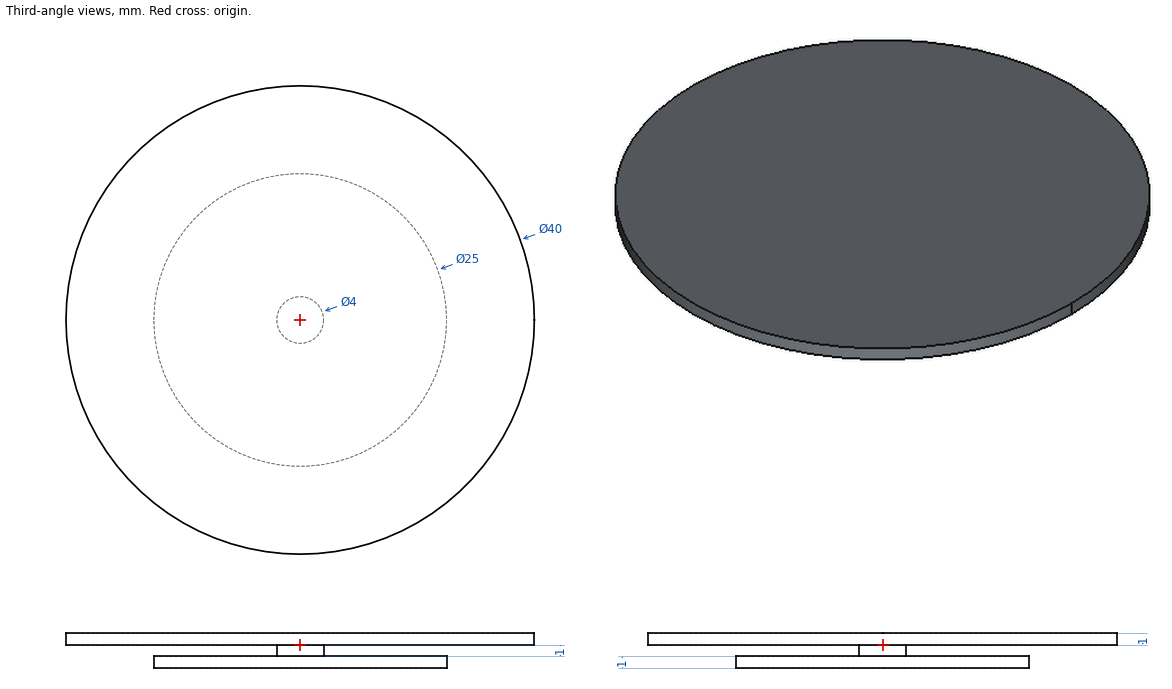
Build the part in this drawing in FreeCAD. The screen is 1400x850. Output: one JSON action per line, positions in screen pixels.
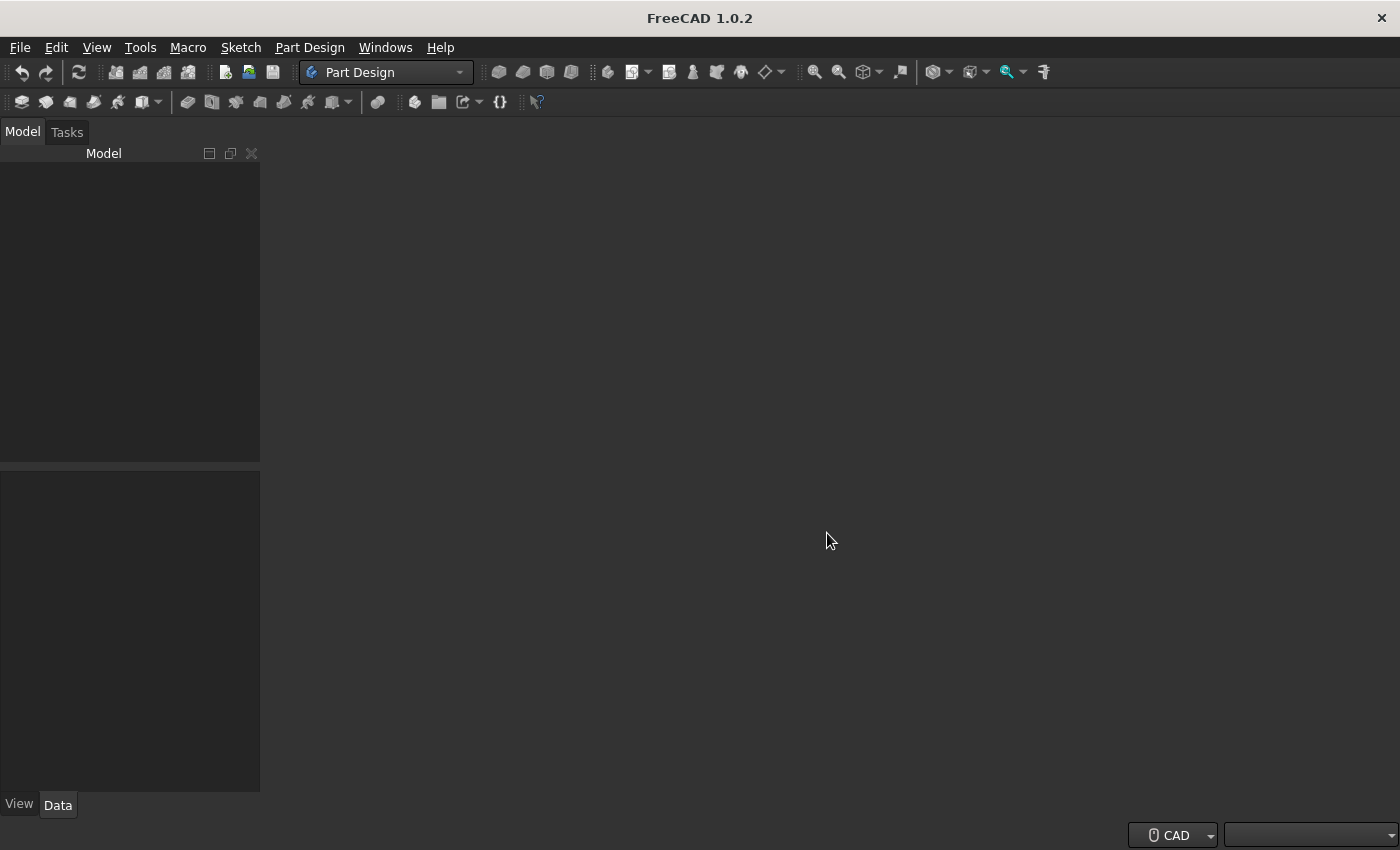
{"action": "key", "text": "ctrl+n"}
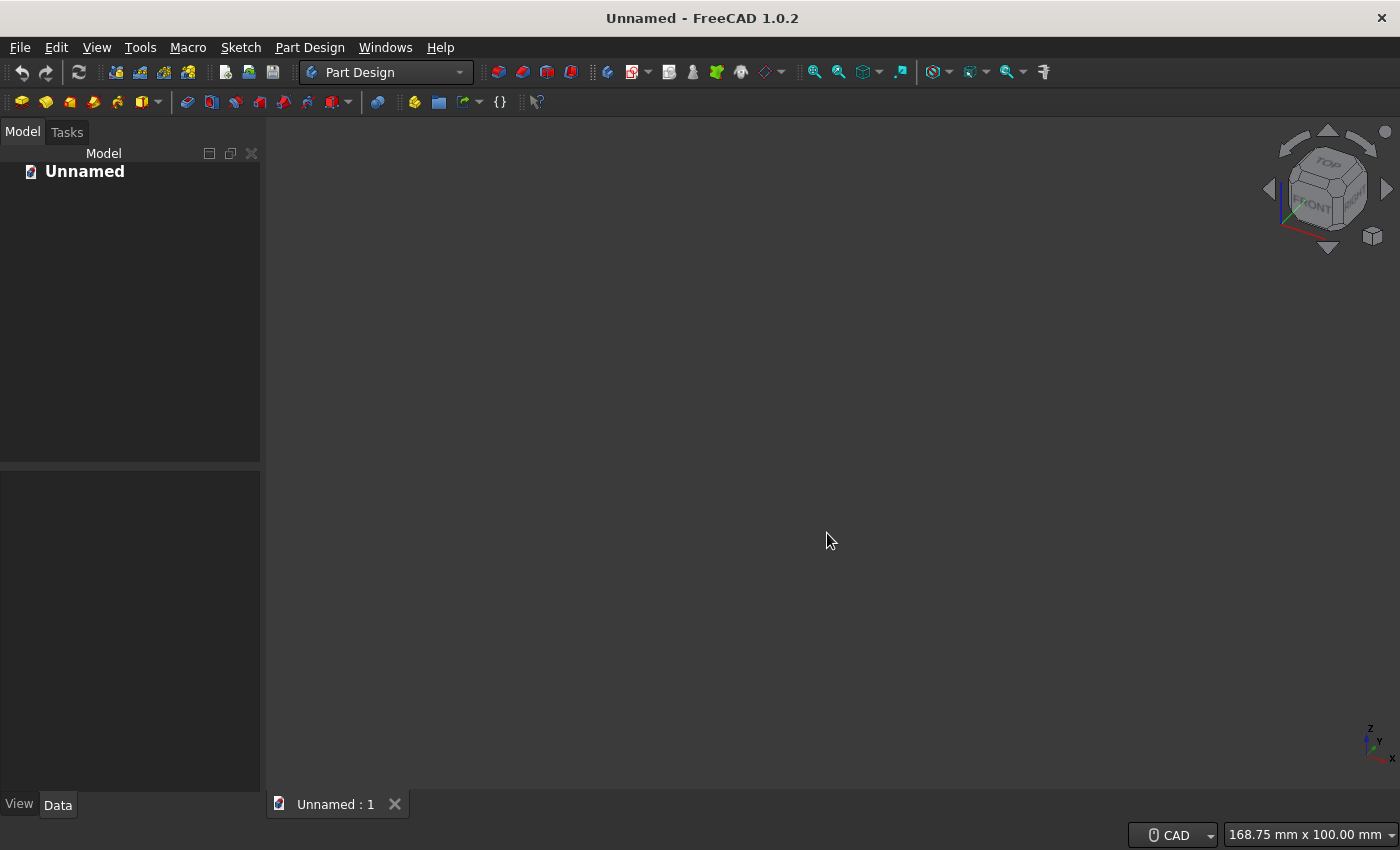
{"action": "left_click", "coordinate": [632, 72]}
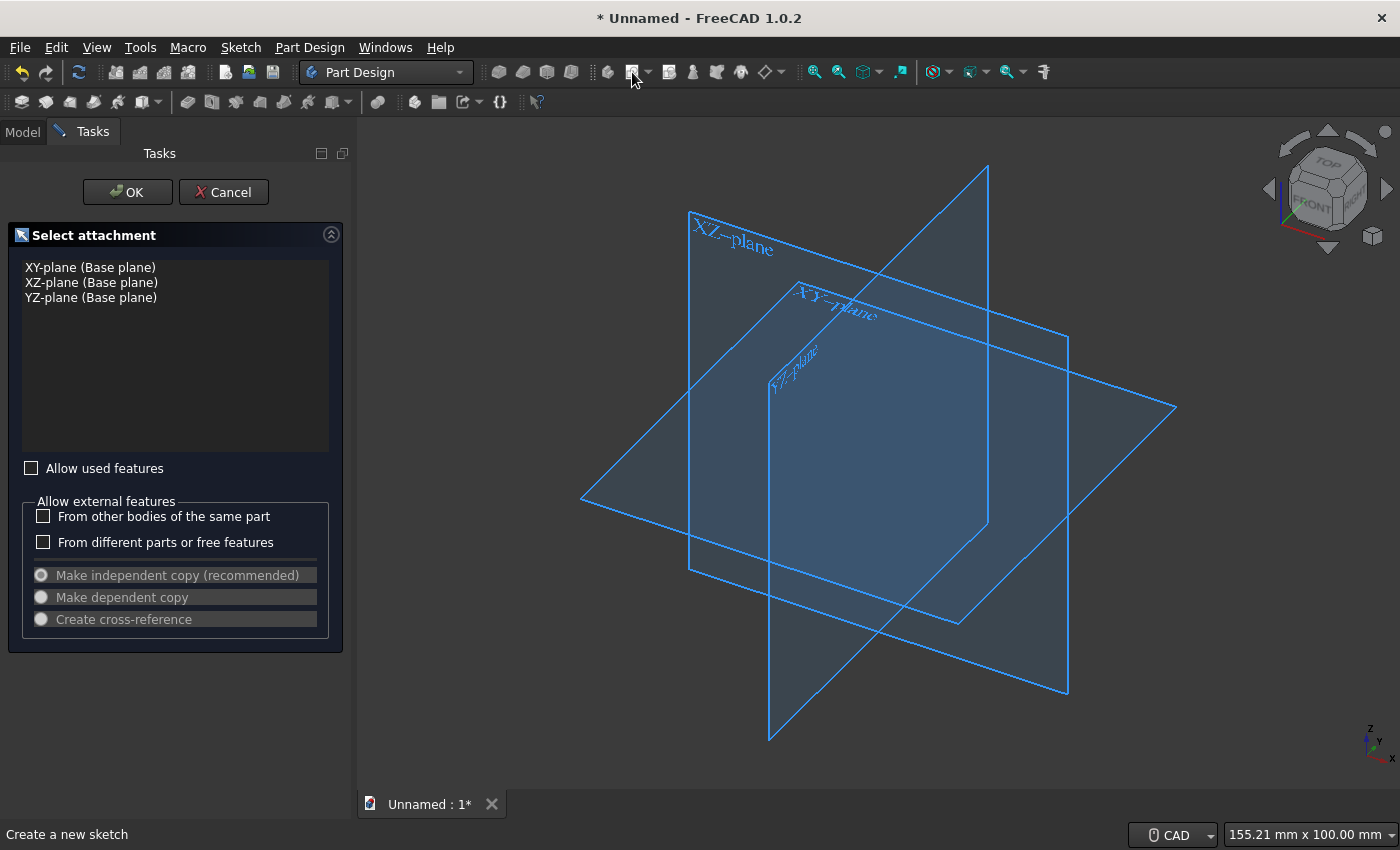
{"action": "left_click", "coordinate": [82, 268]}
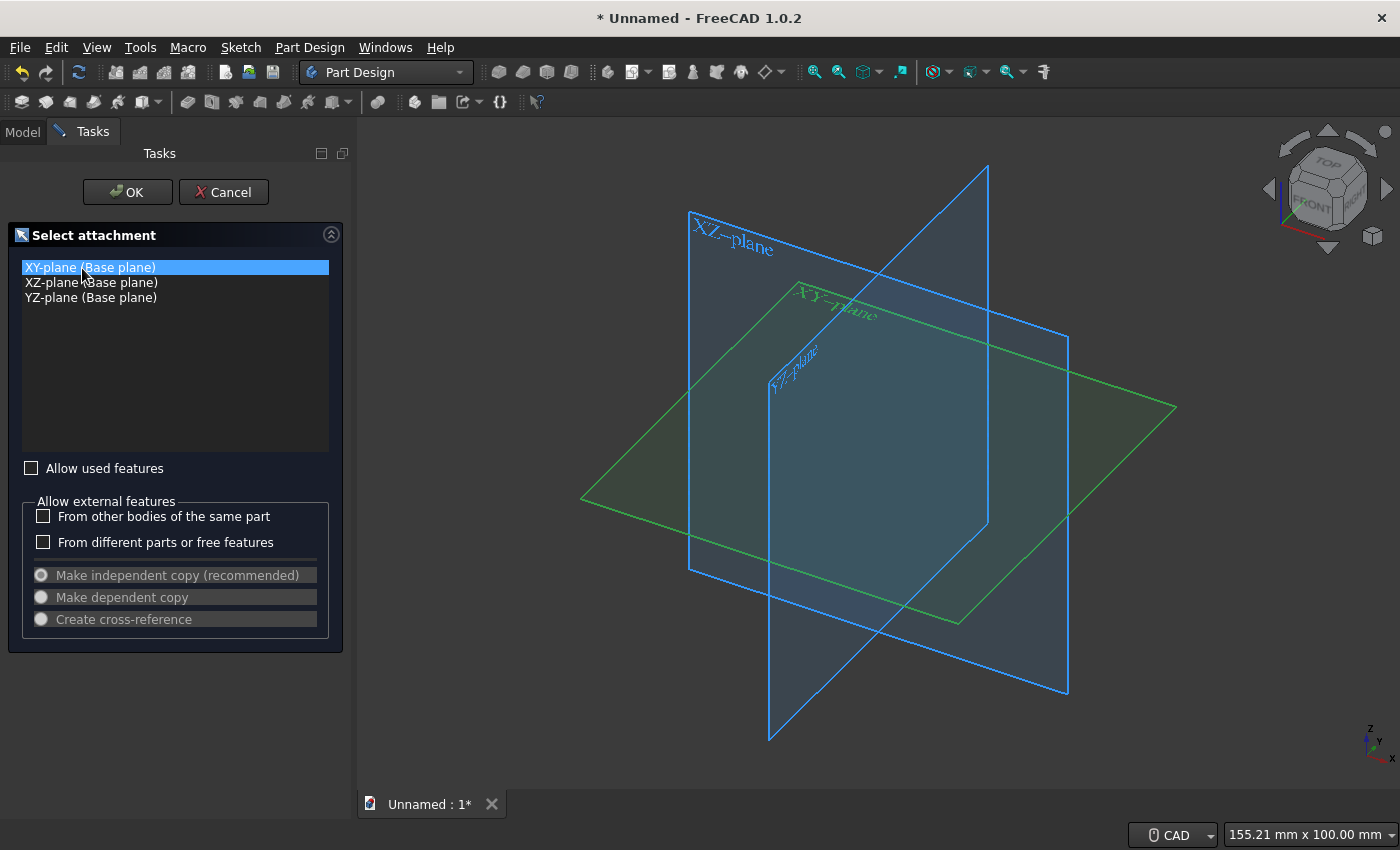
{"action": "left_click", "coordinate": [128, 192]}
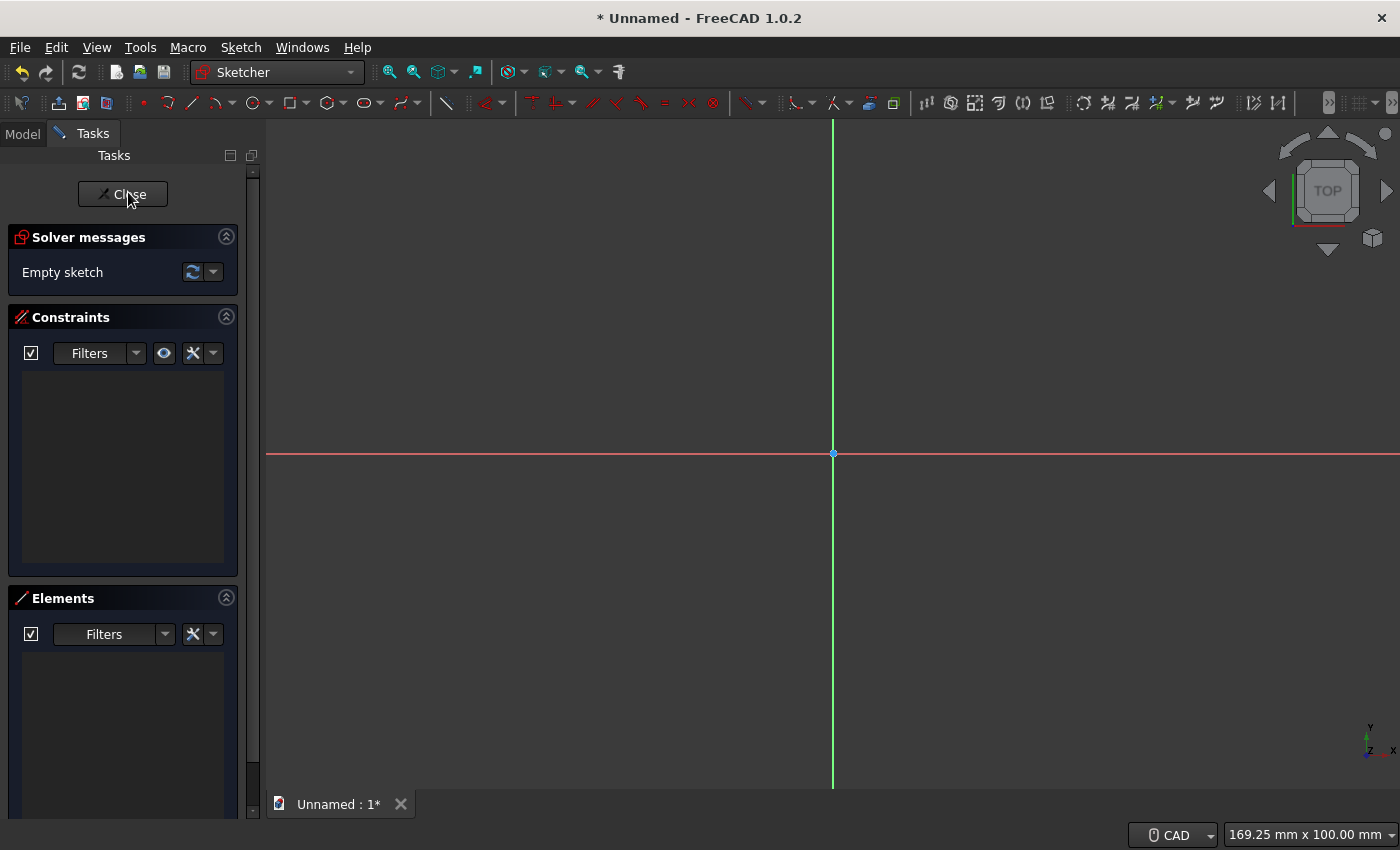
{"action": "scroll", "coordinate": [972, 454], "scroll_direction": "up", "scroll_amount": 2}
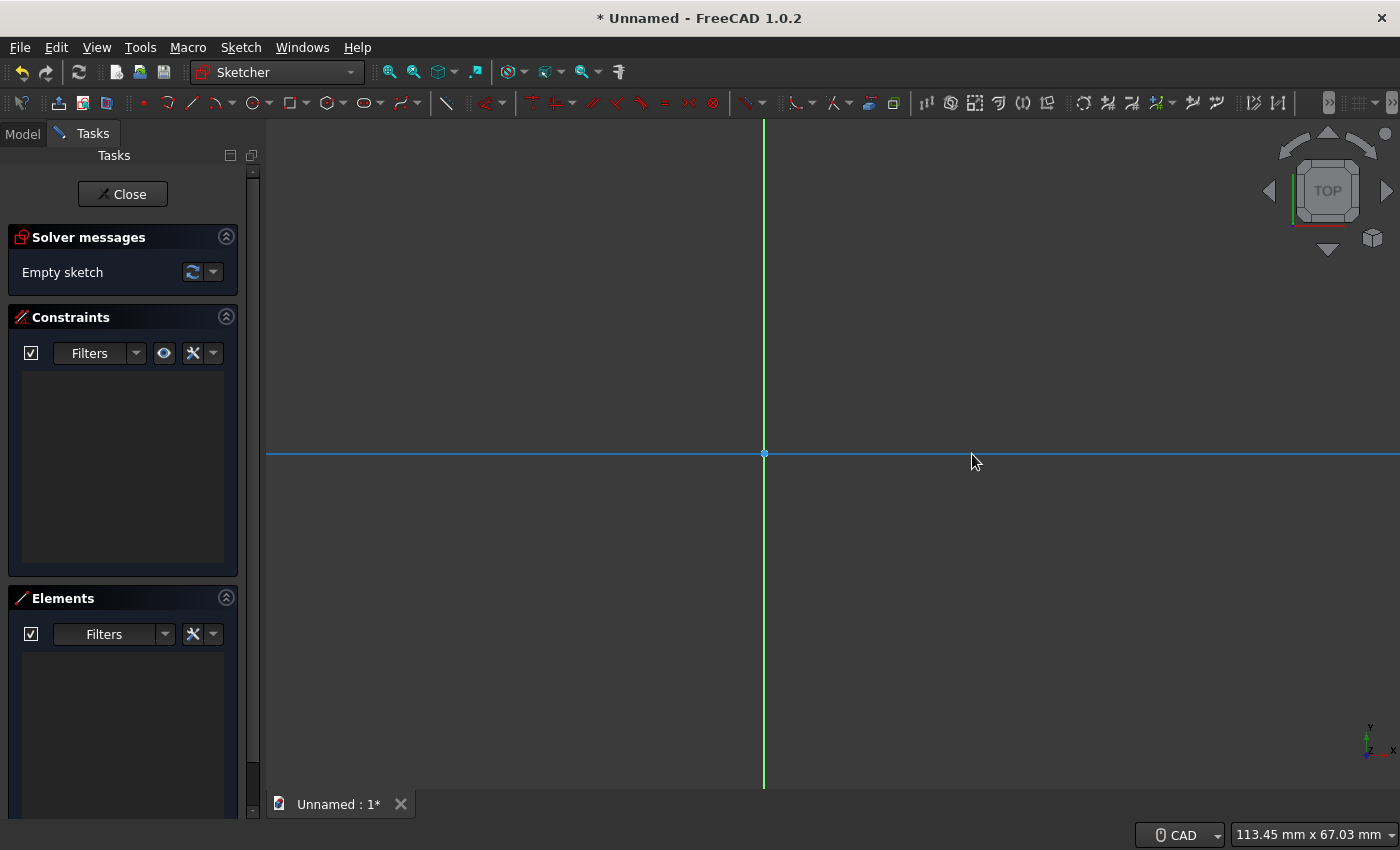
{"action": "key", "text": "g c"}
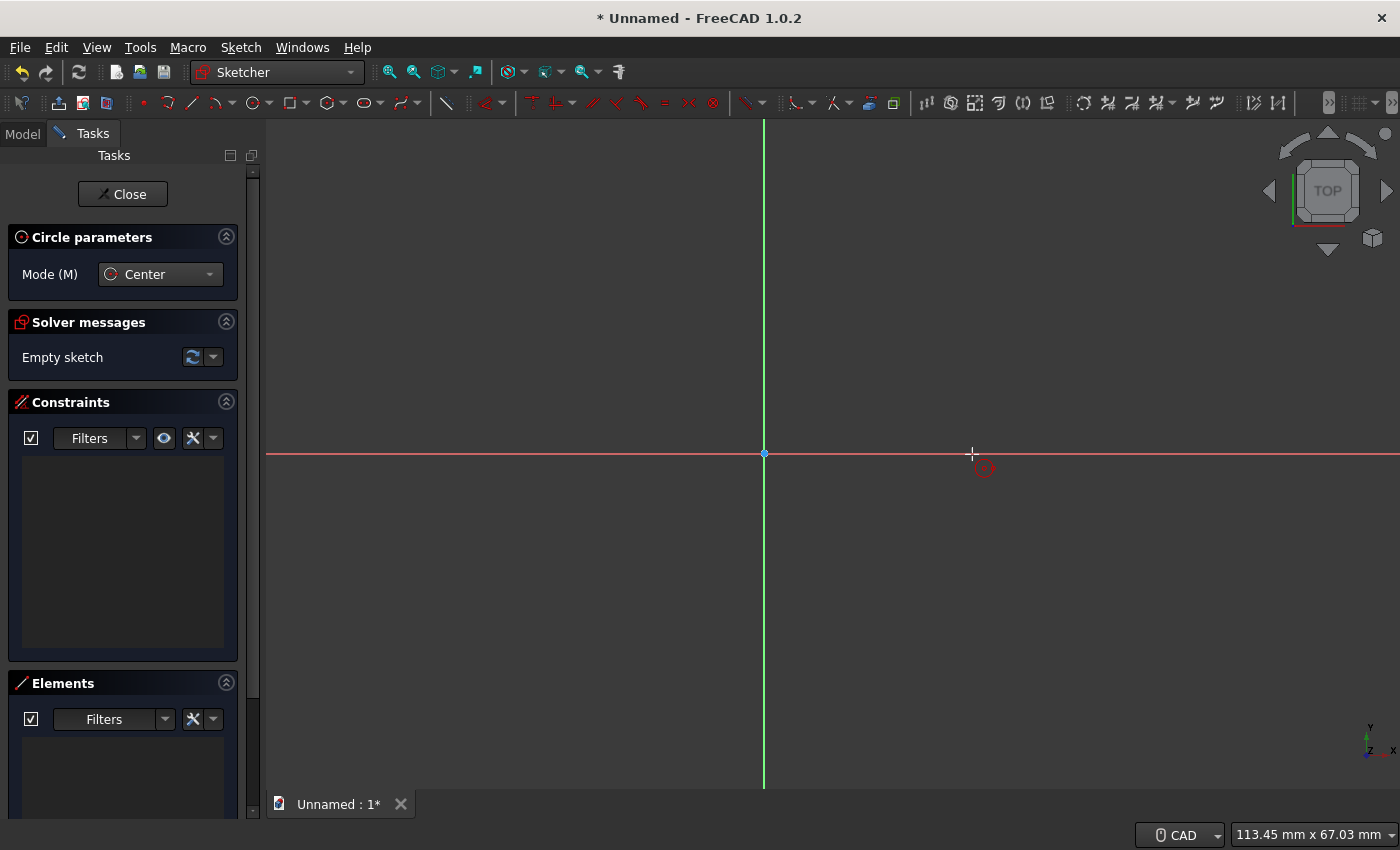
{"action": "left_click", "coordinate": [764, 454]}
{"action": "left_click", "coordinate": [906, 312]}
{"action": "key", "text": "Escape"}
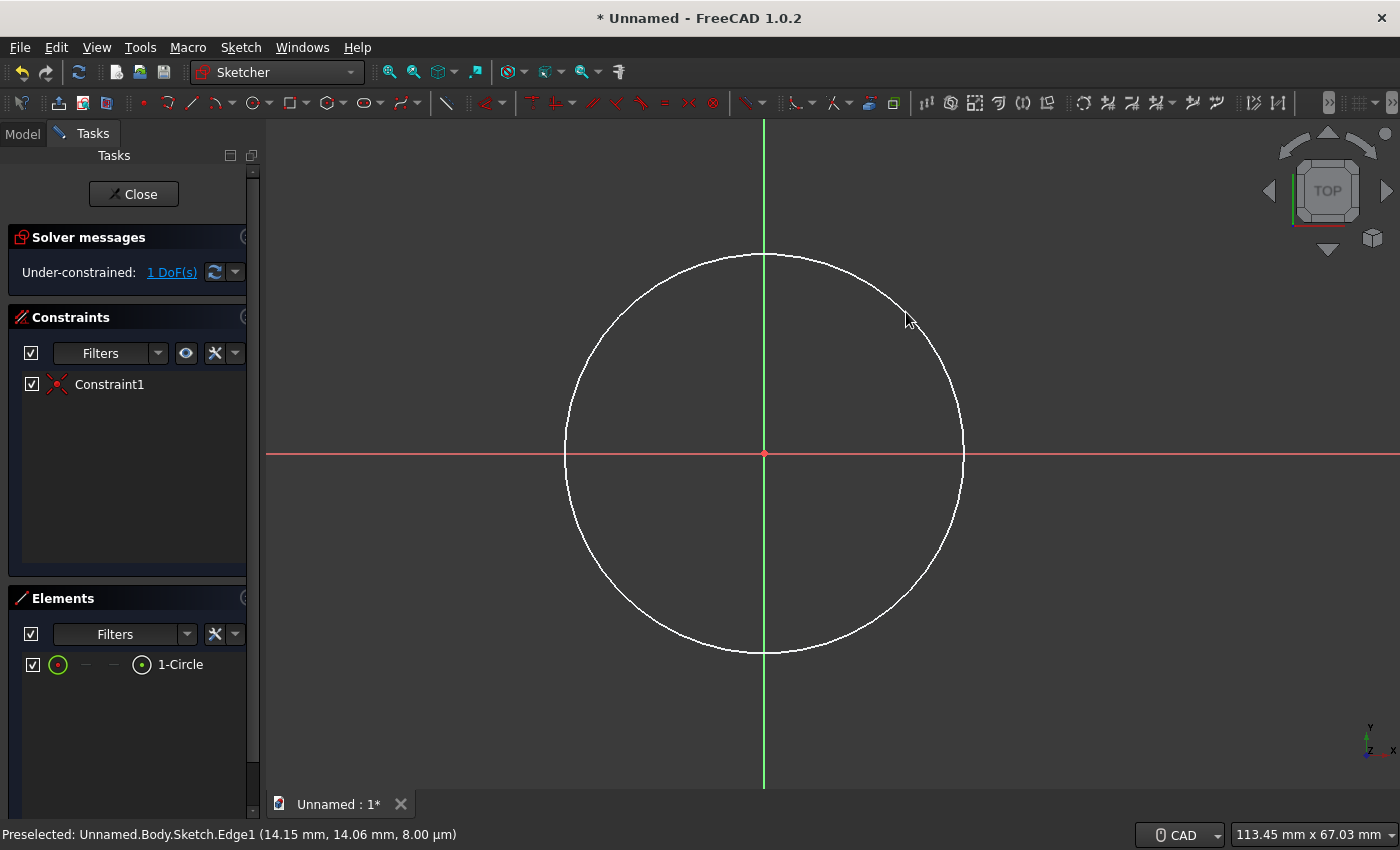
{"action": "left_click", "coordinate": [486, 104]}